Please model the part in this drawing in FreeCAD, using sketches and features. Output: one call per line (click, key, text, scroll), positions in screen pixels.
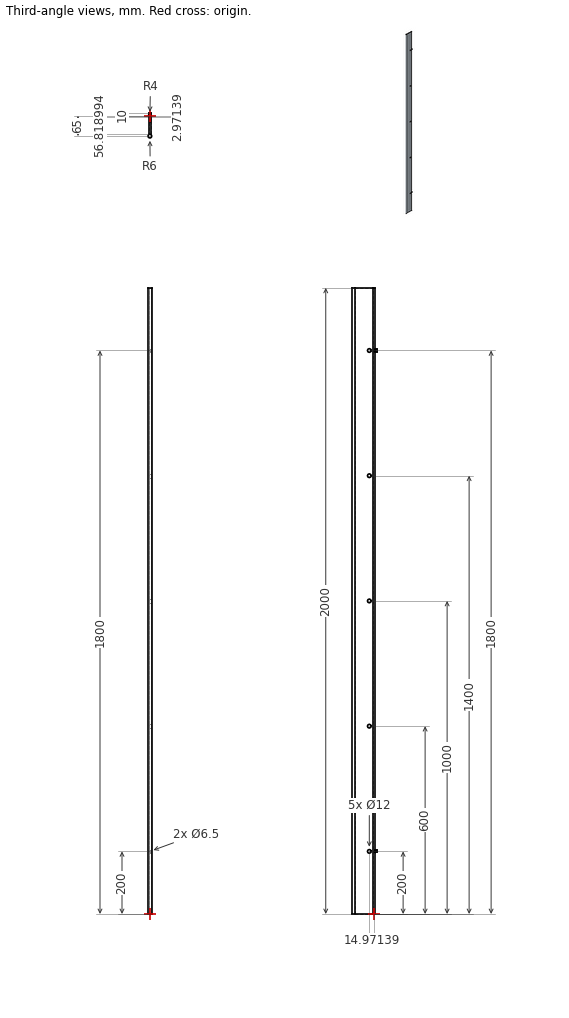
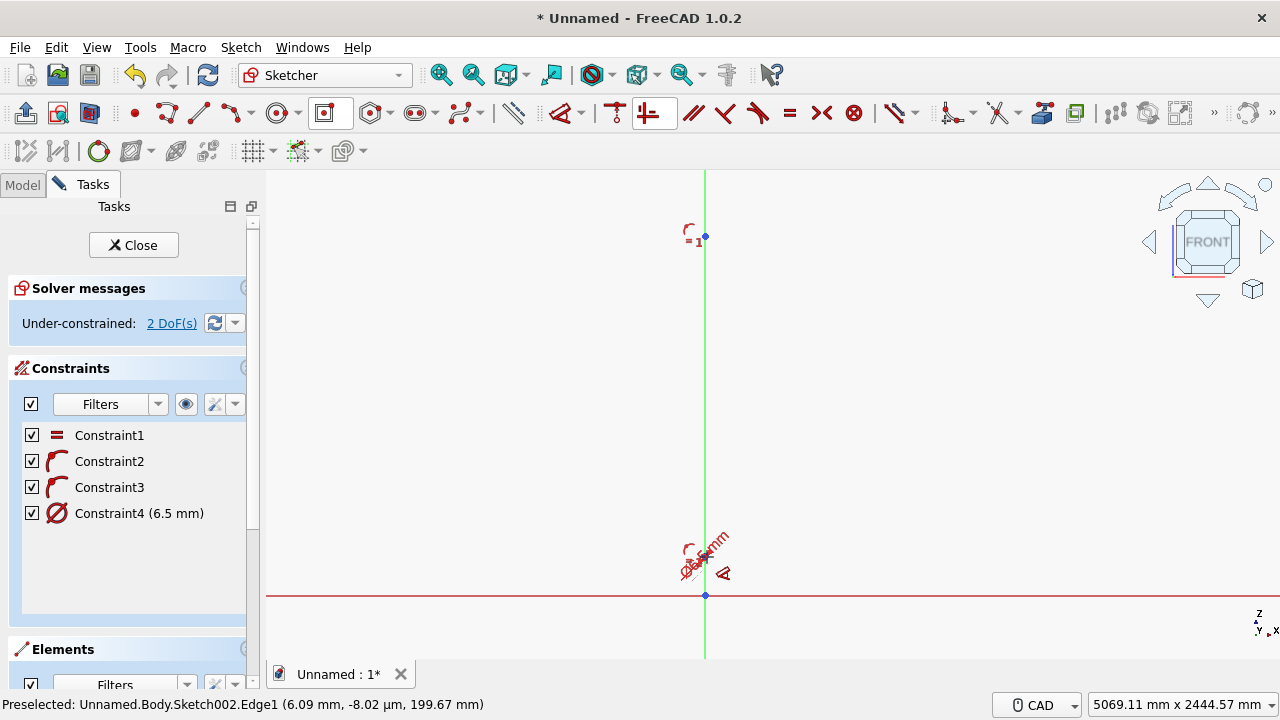
click(705, 557)
click(739, 576)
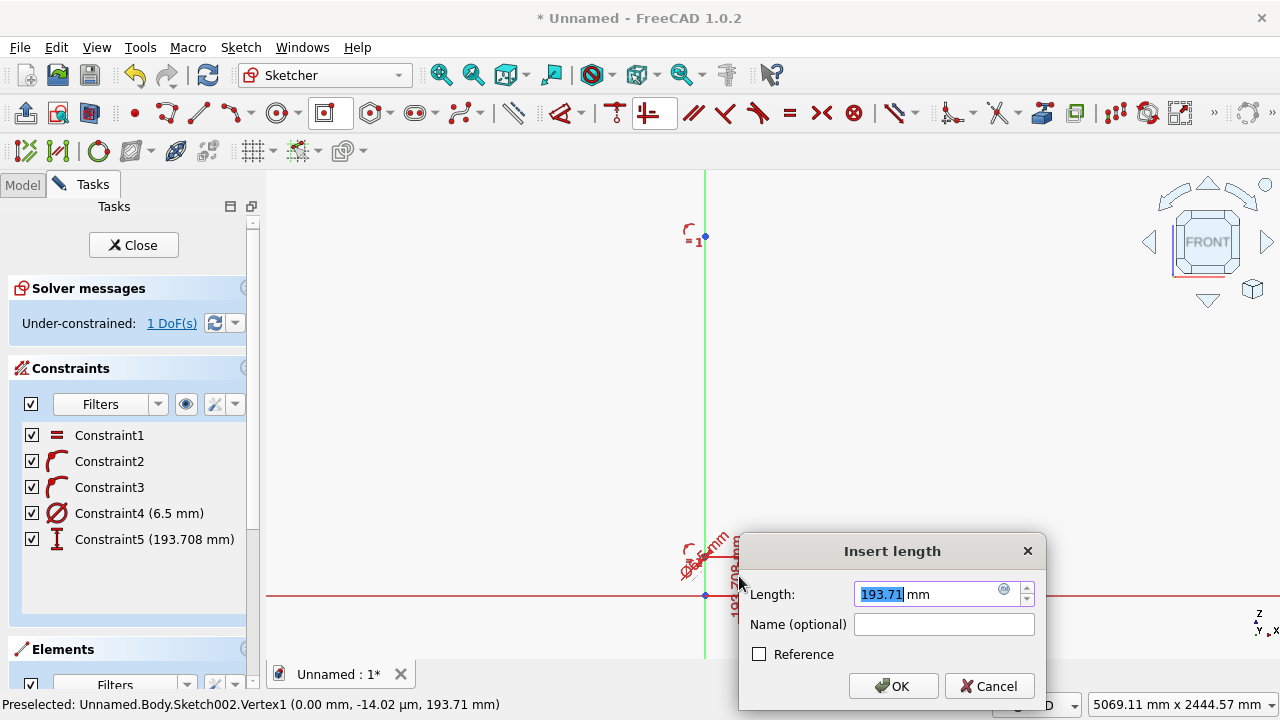
text(200)
key(Return)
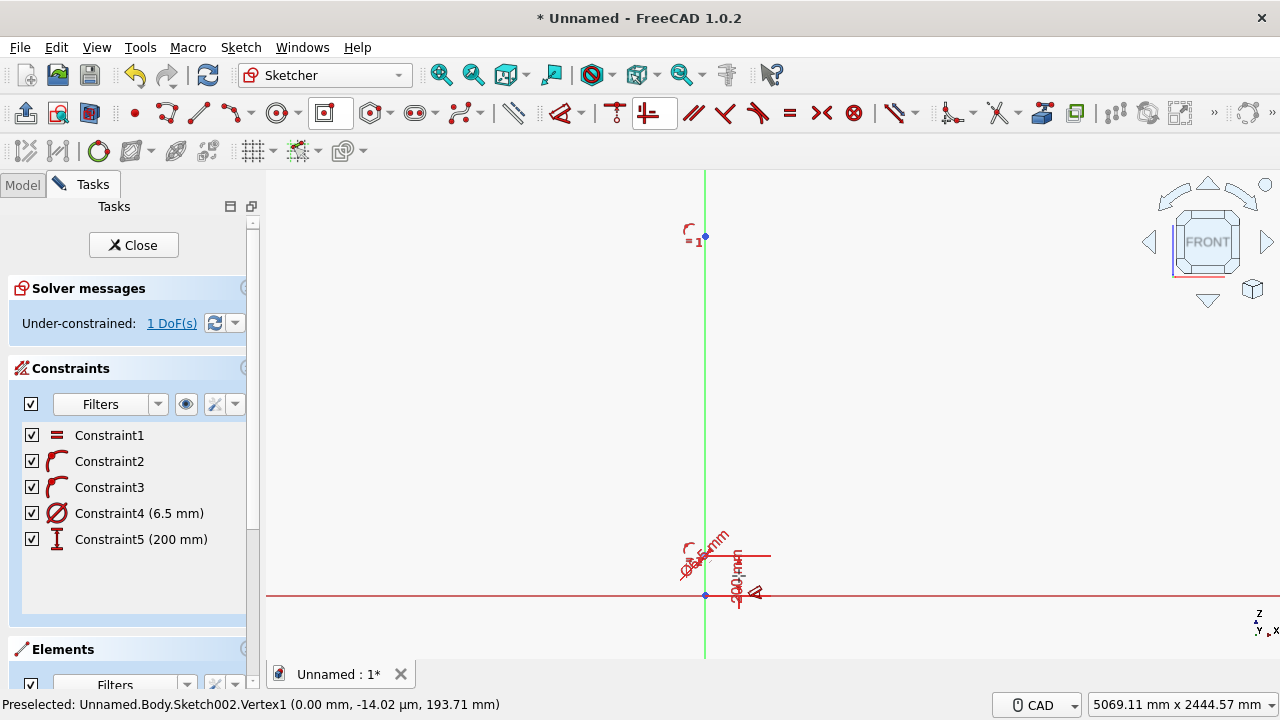
click(705, 237)
click(739, 416)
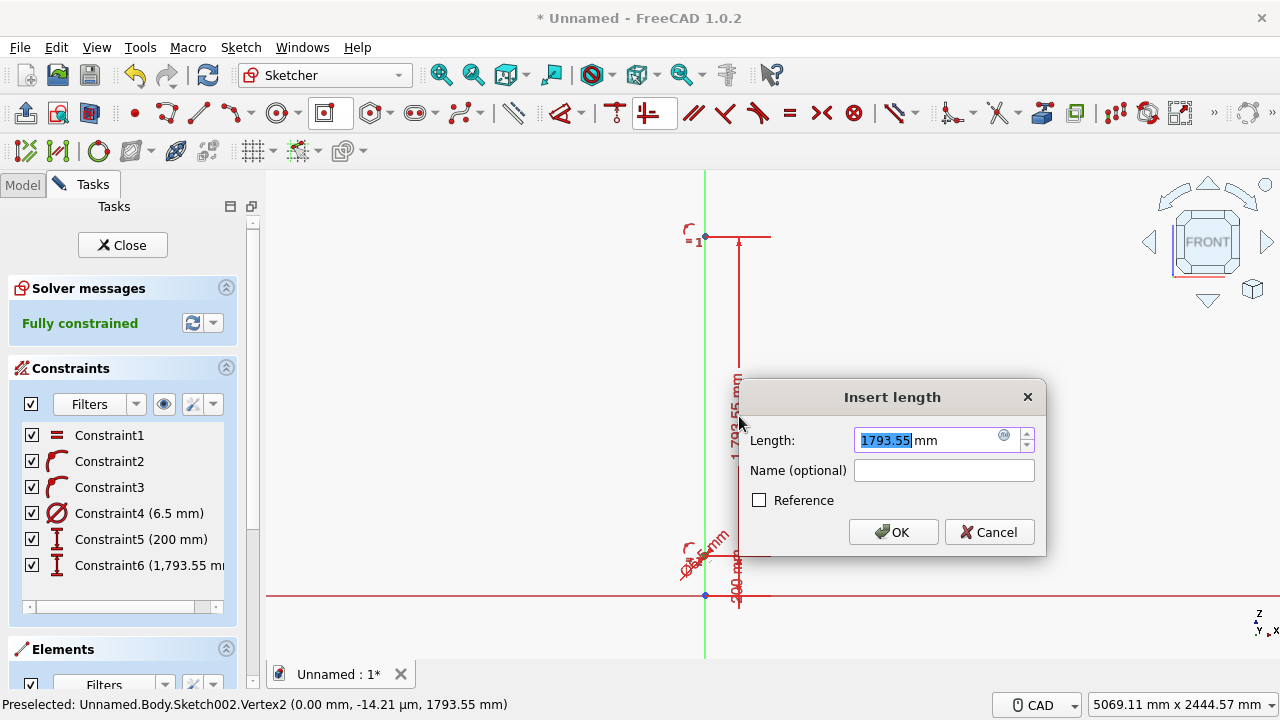
text(1800)
key(Return)
key(Escape)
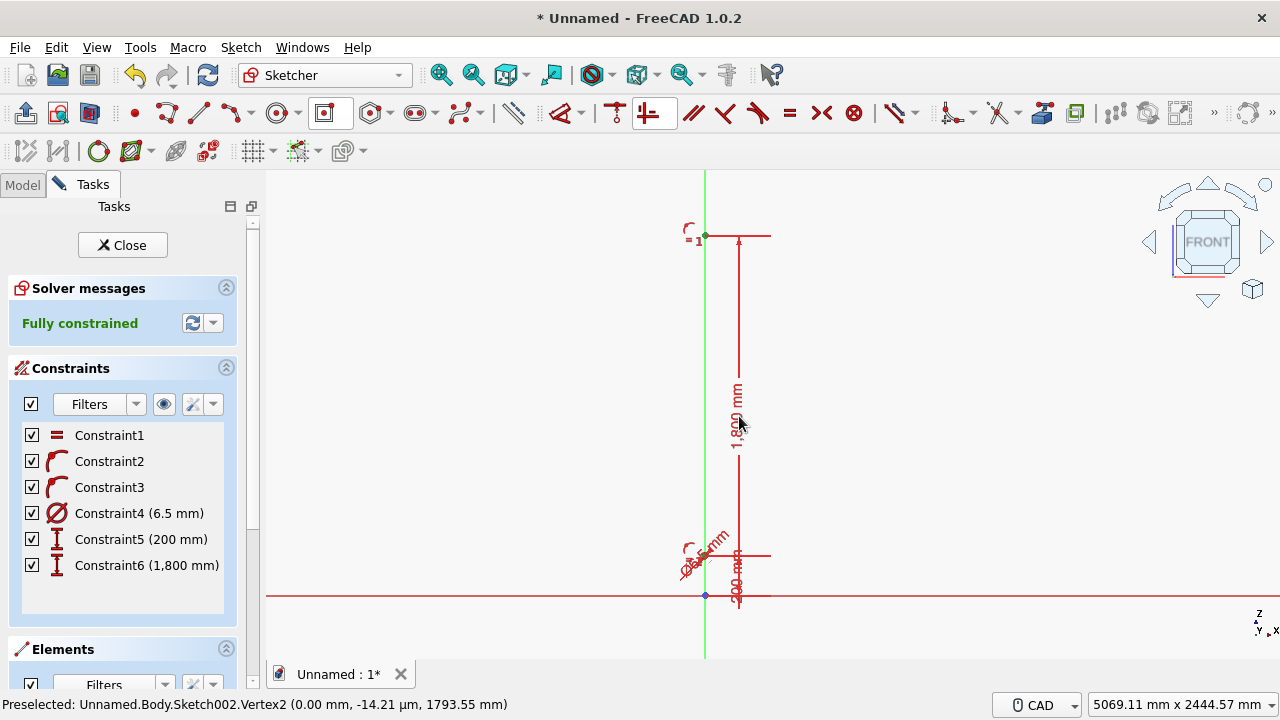
click(123, 245)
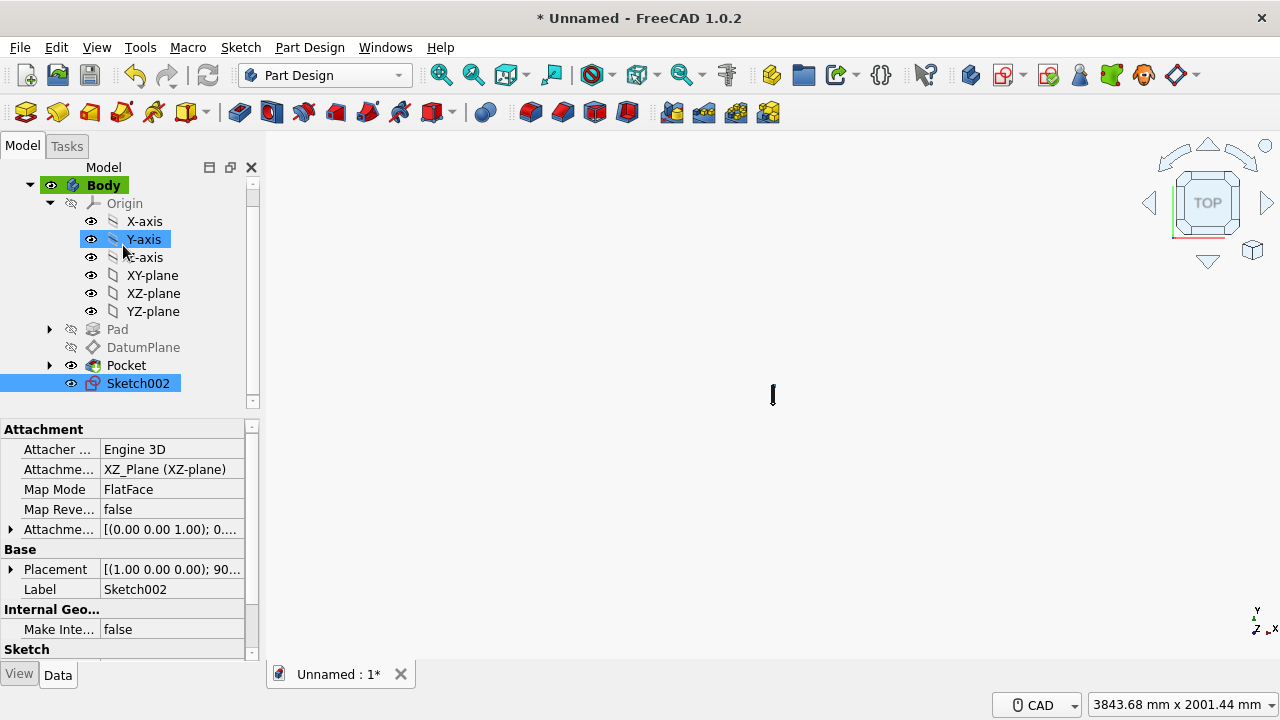
click(26, 112)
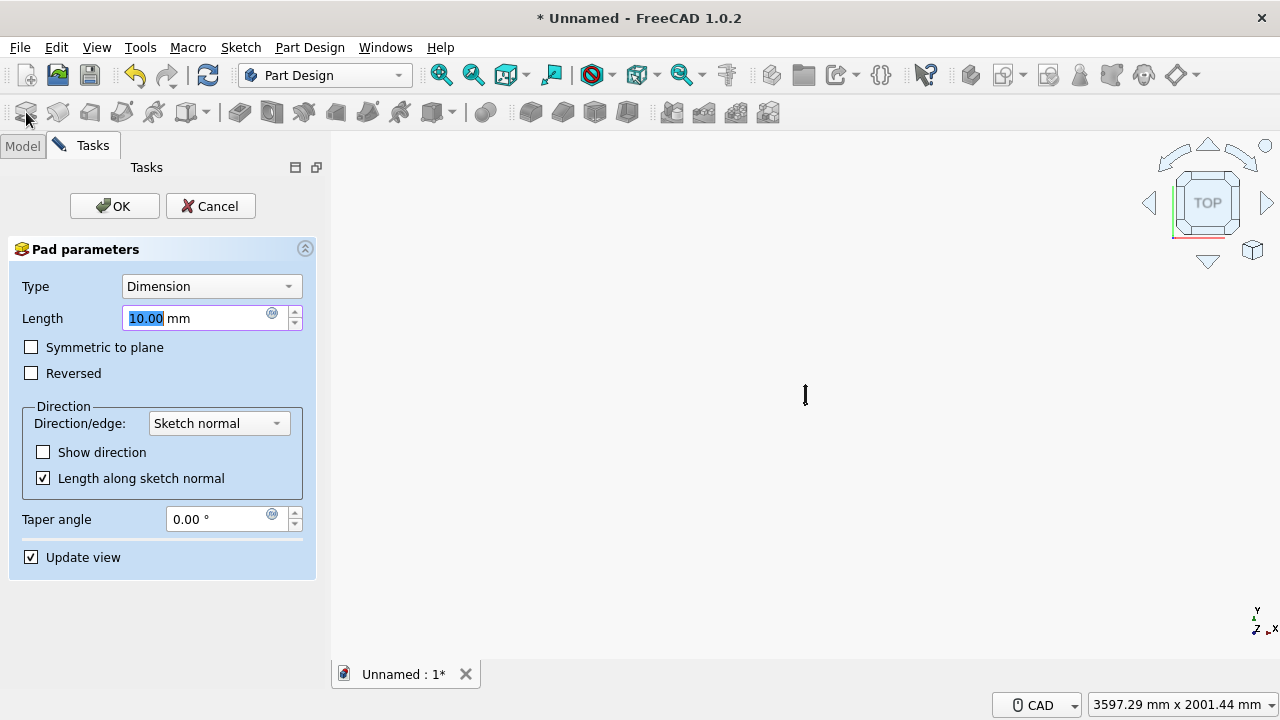
text(10)
key(Tab)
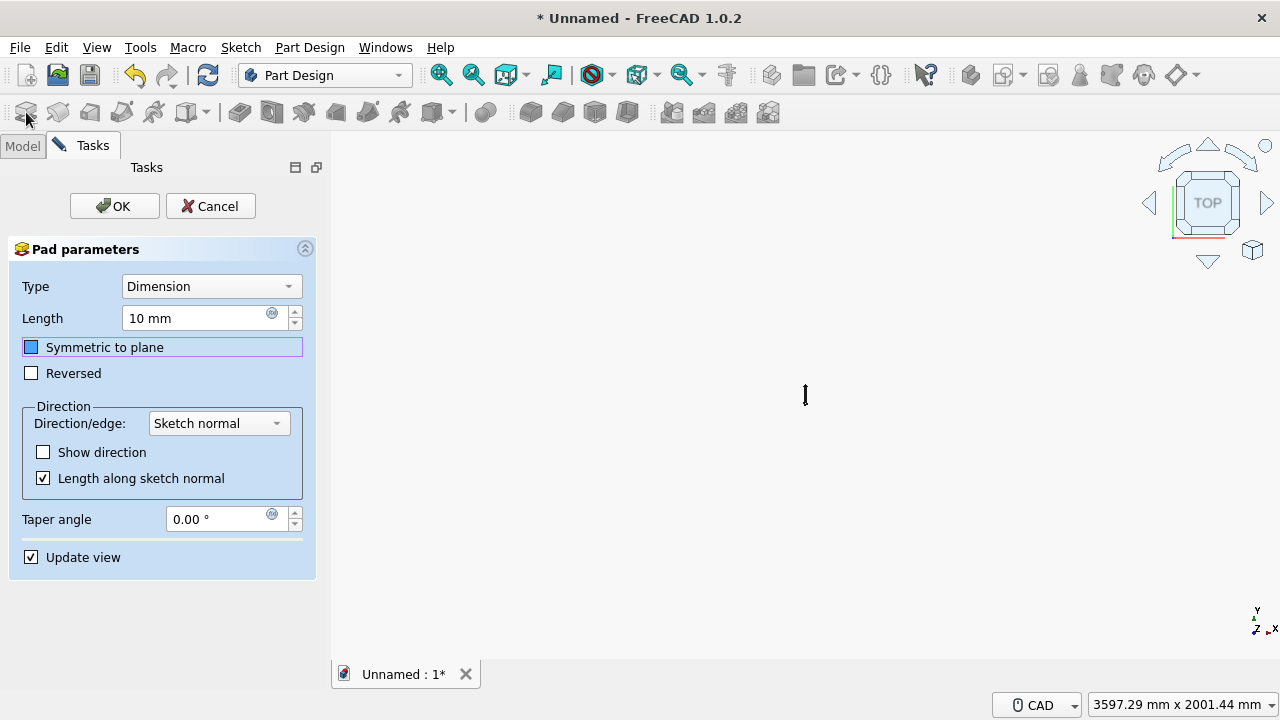
click(30, 373)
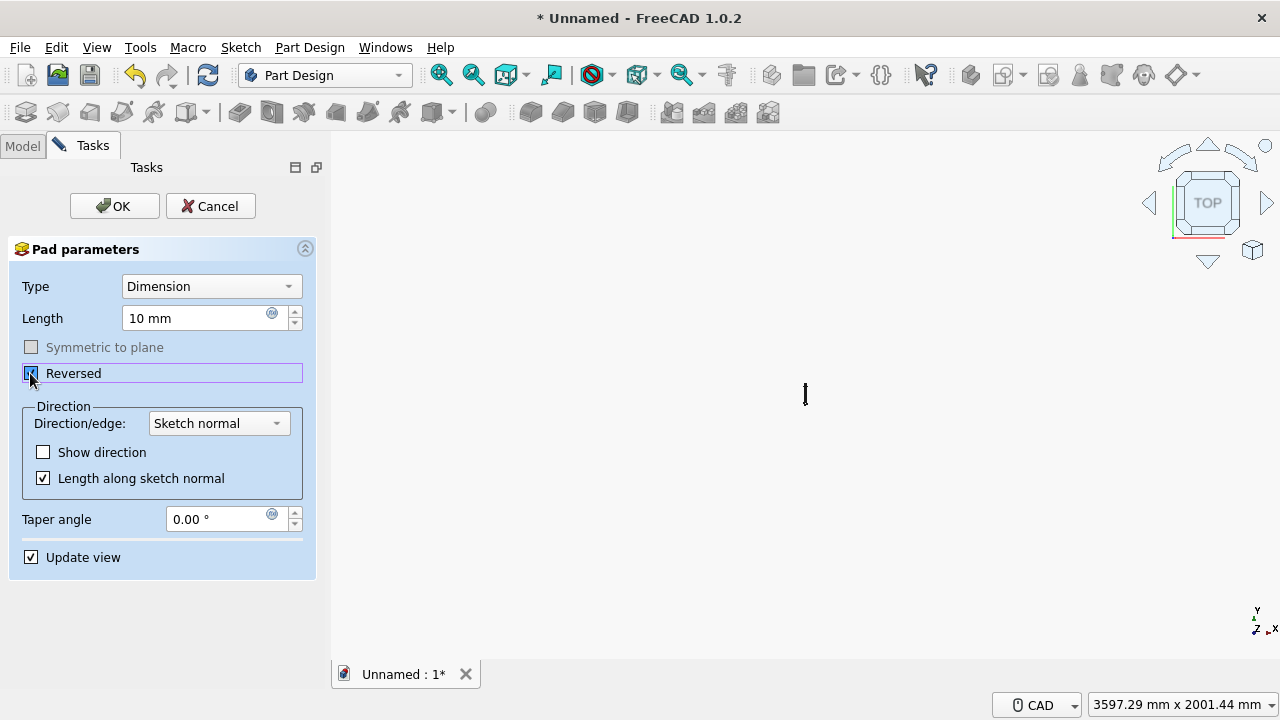
click(115, 206)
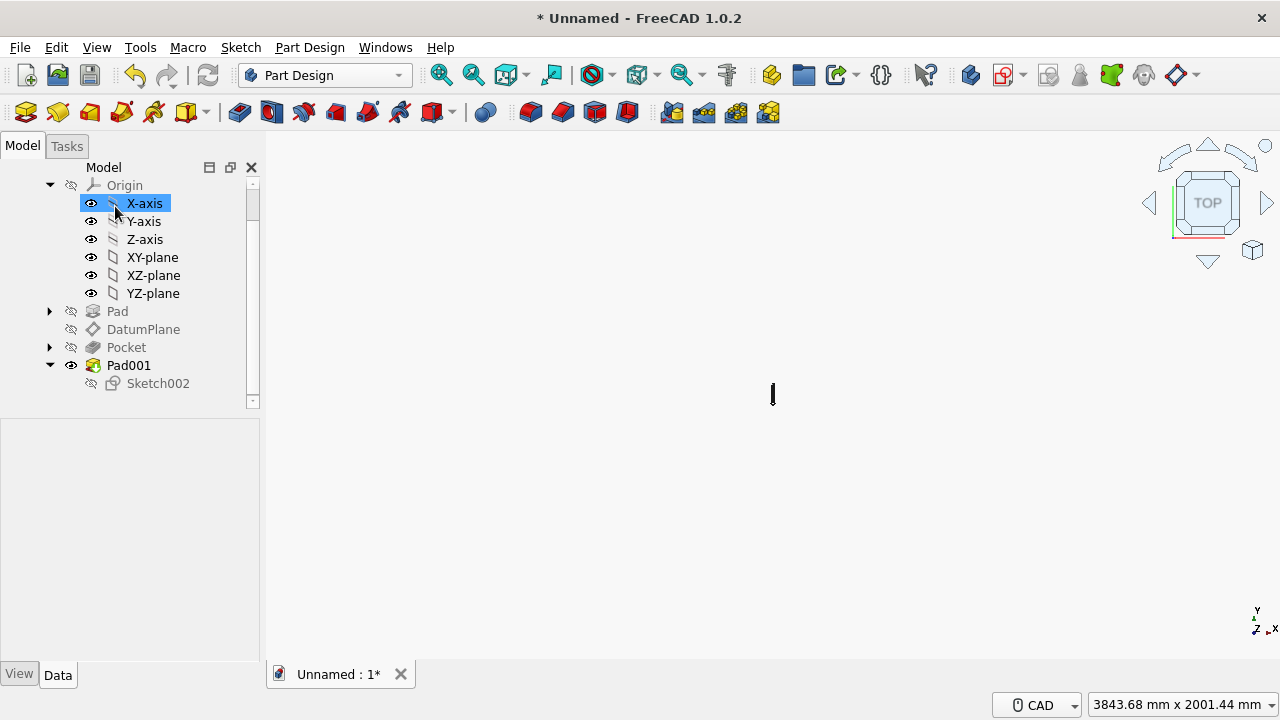
key(0)